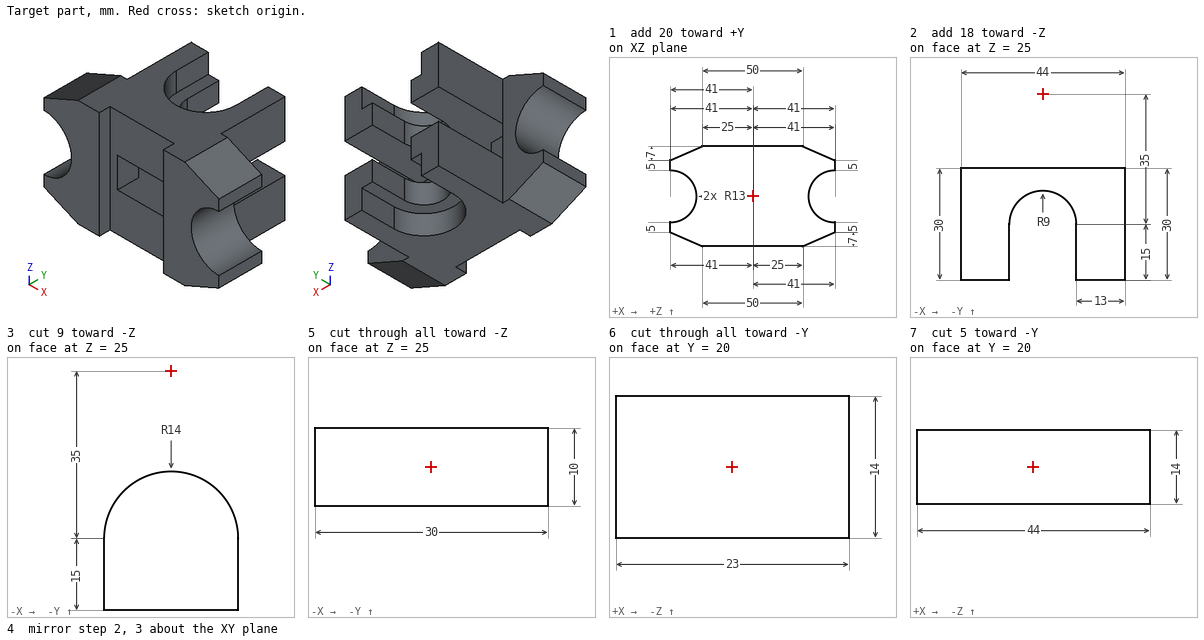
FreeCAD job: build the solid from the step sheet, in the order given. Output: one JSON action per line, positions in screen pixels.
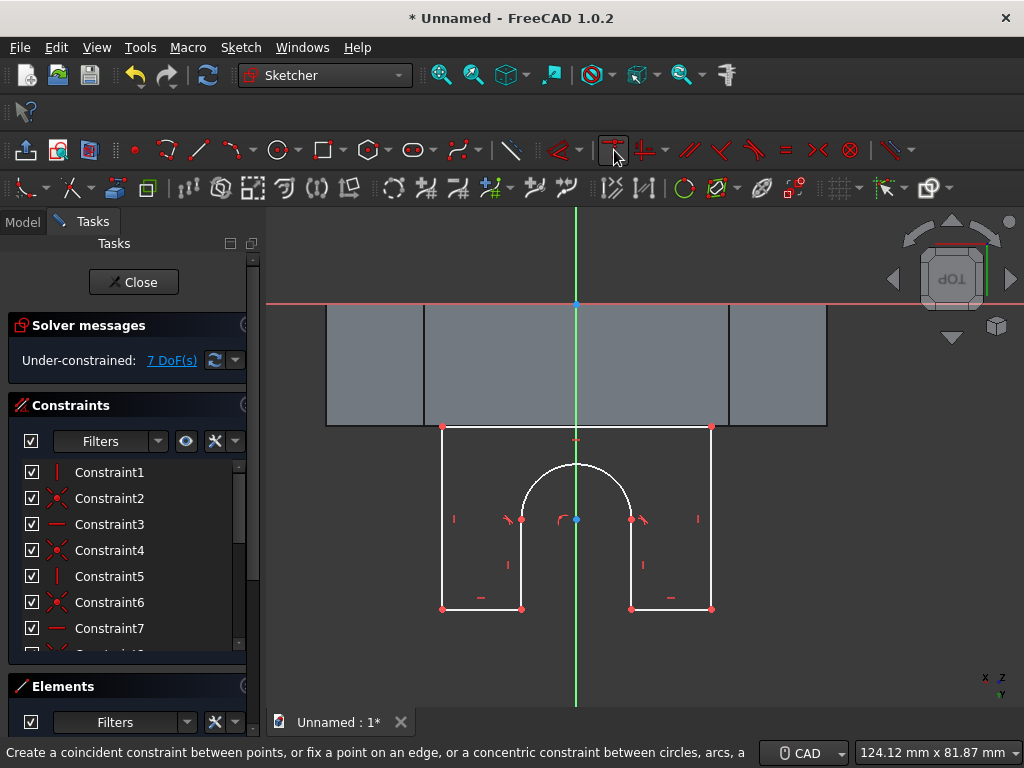
{"action": "left_click", "coordinate": [558, 150]}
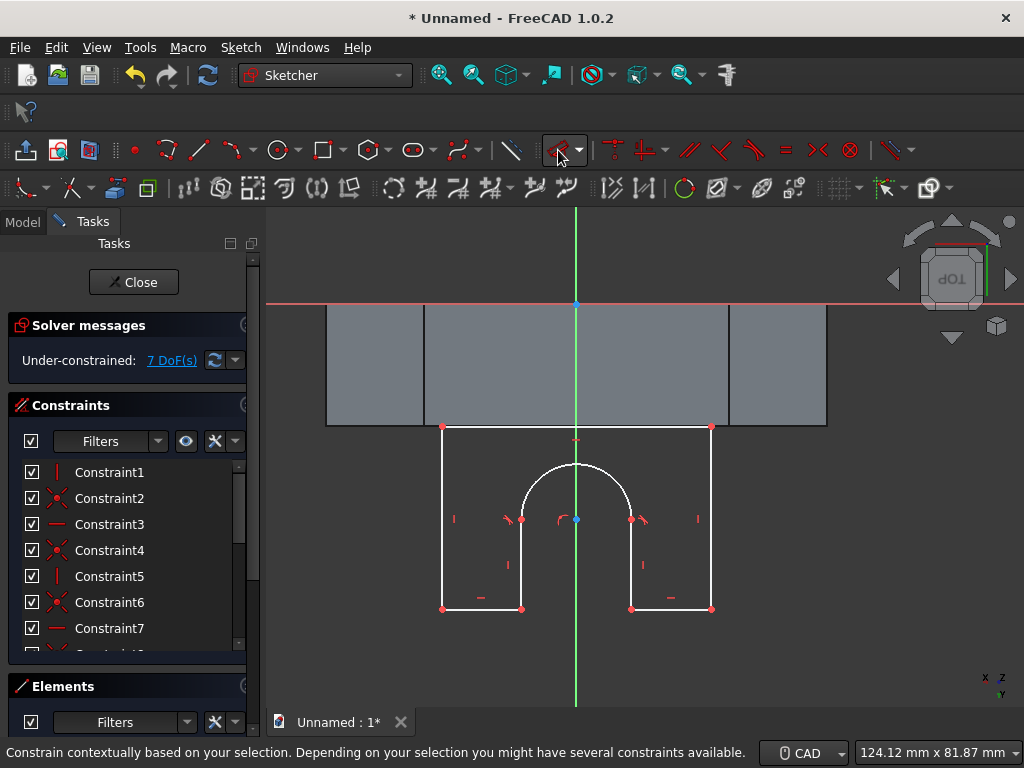
{"action": "left_click", "coordinate": [609, 475]}
{"action": "left_click", "coordinate": [628, 449]}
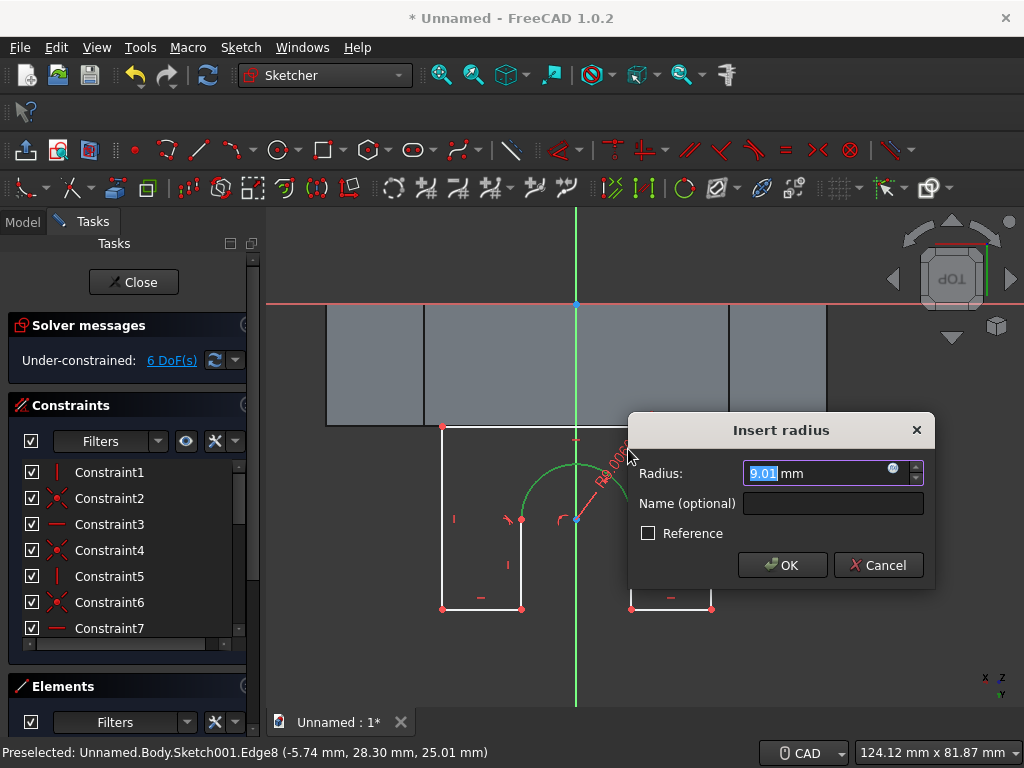
{"action": "type", "text": "9"}
{"action": "key", "text": "Return"}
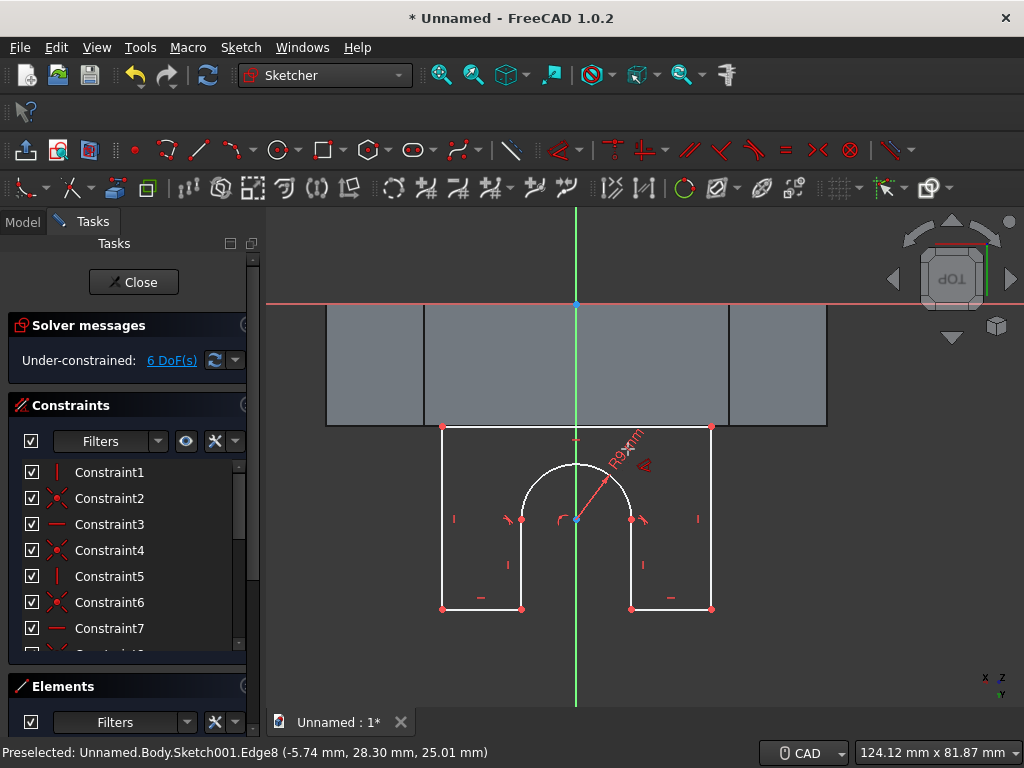
{"action": "left_click", "coordinate": [631, 547]}
{"action": "left_click", "coordinate": [665, 565]}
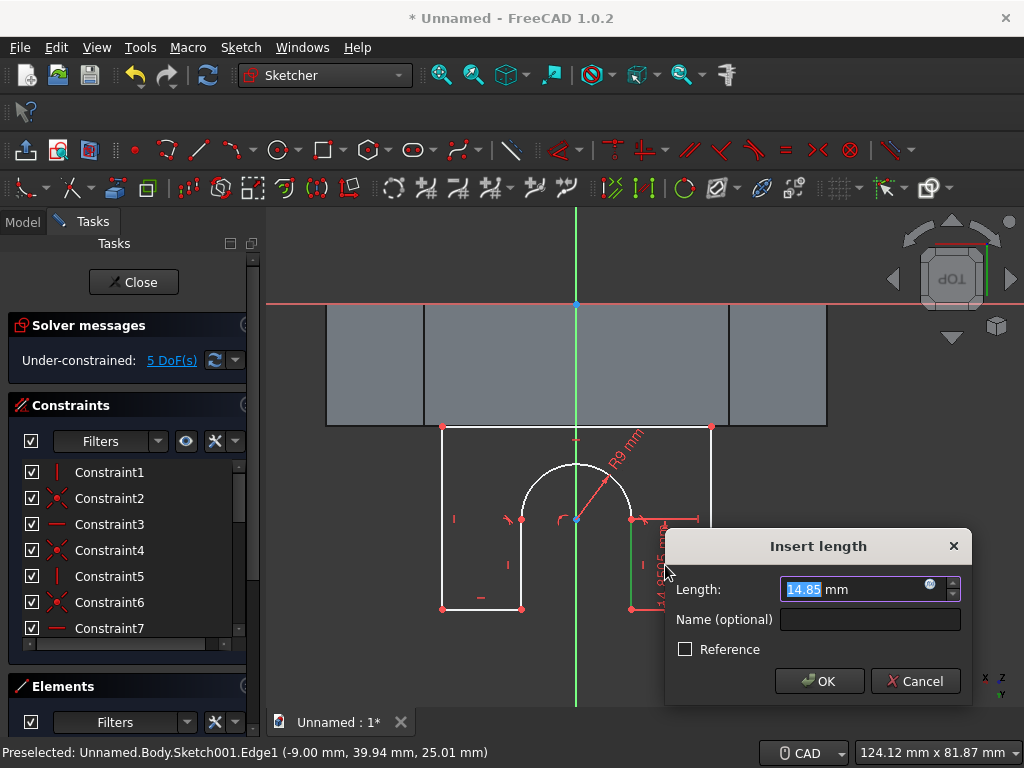
{"action": "type", "text": "15"}
{"action": "key", "text": "Return"}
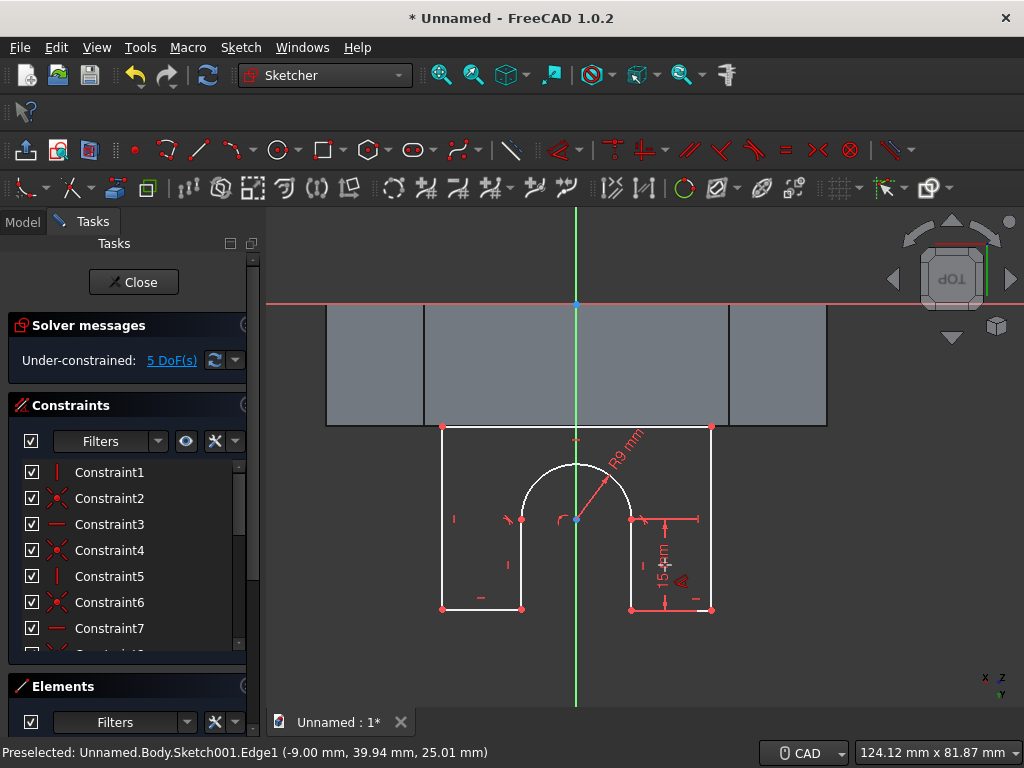
{"action": "left_click", "coordinate": [655, 611]}
{"action": "left_click", "coordinate": [671, 645]}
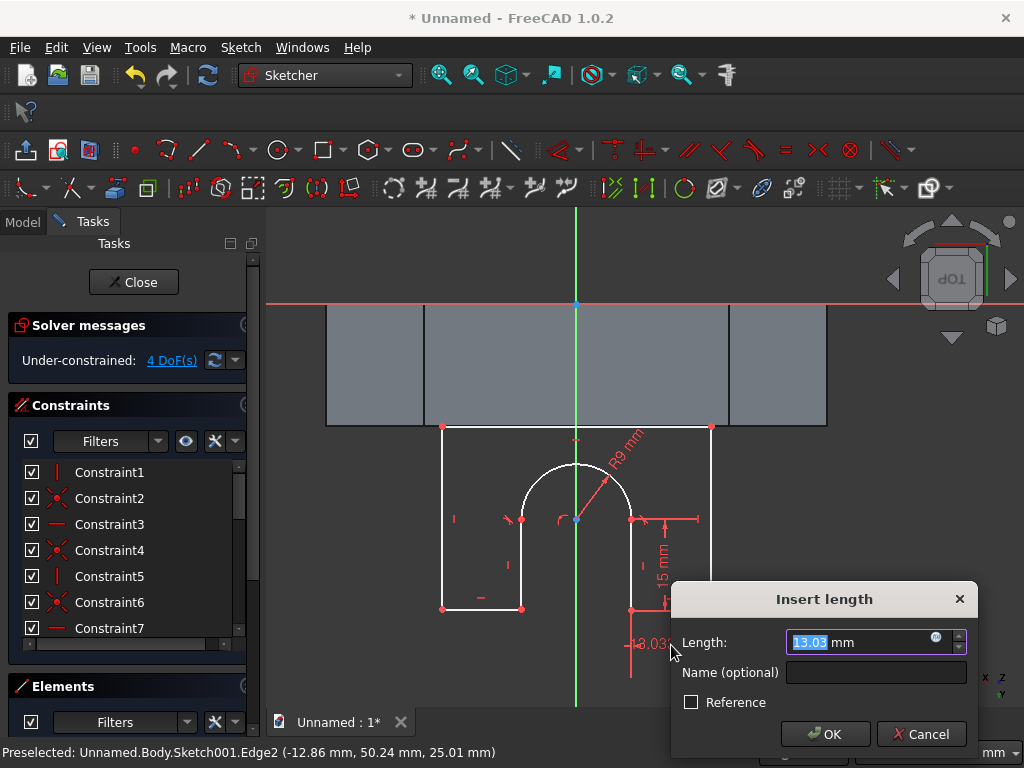
{"action": "type", "text": "13"}
{"action": "key", "text": "Return"}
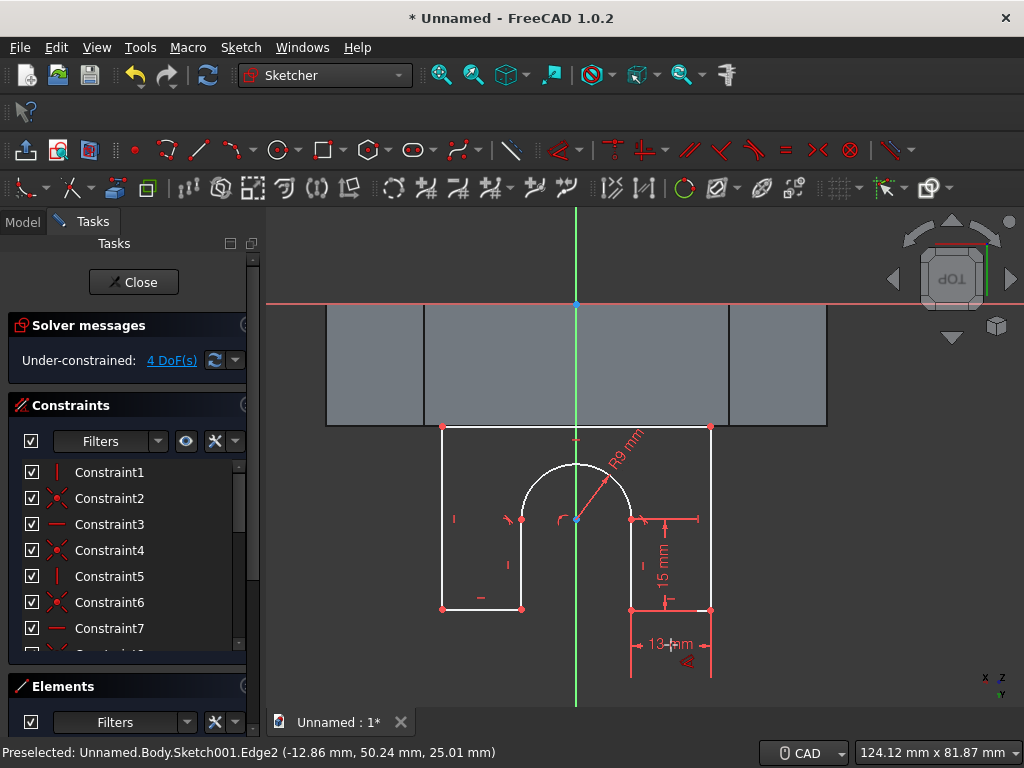
{"action": "left_click", "coordinate": [711, 556]}
{"action": "left_click", "coordinate": [745, 519]}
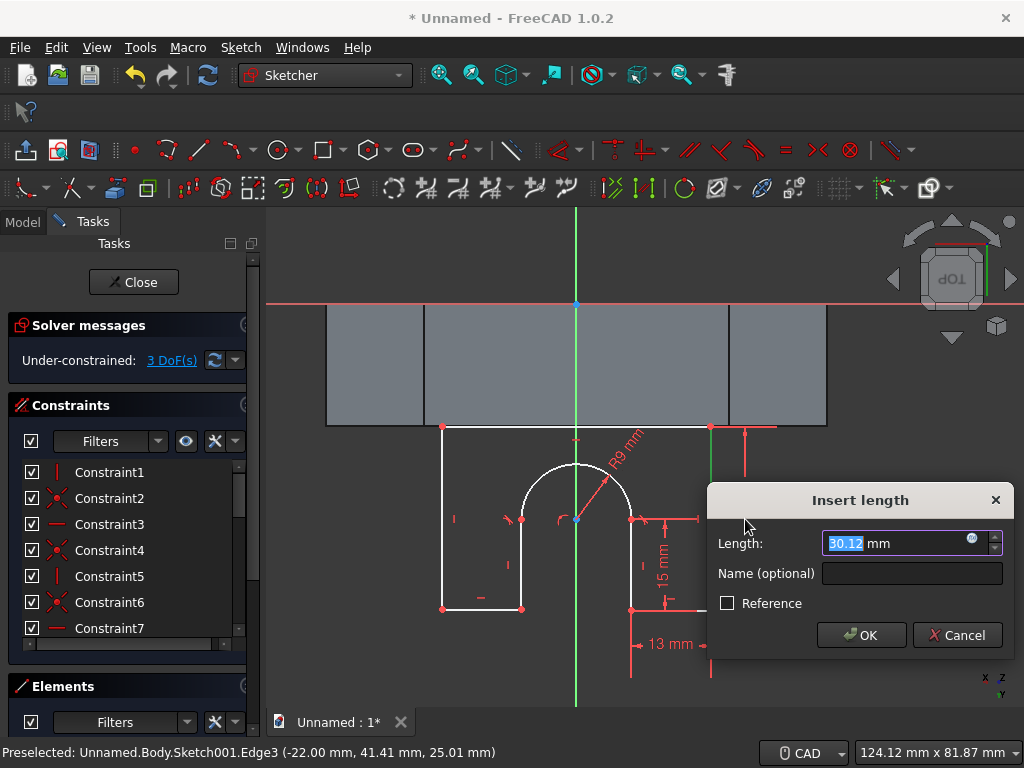
{"action": "type", "text": "30"}
{"action": "key", "text": "Return"}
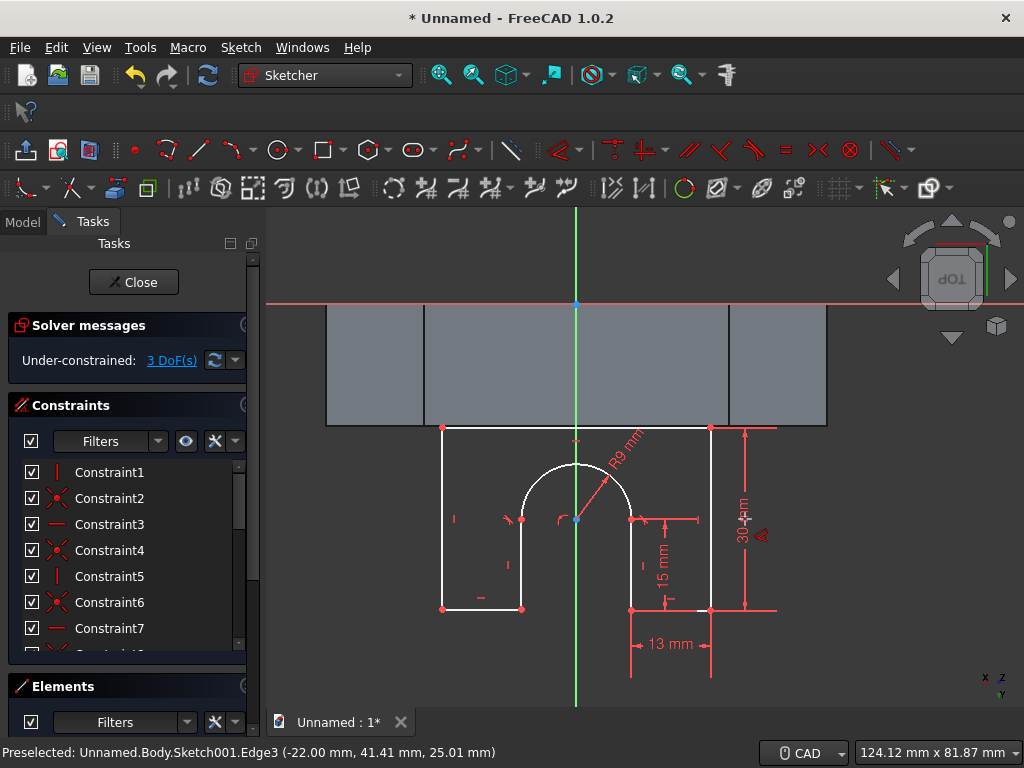
{"action": "left_click", "coordinate": [630, 428]}
{"action": "left_click", "coordinate": [515, 394]}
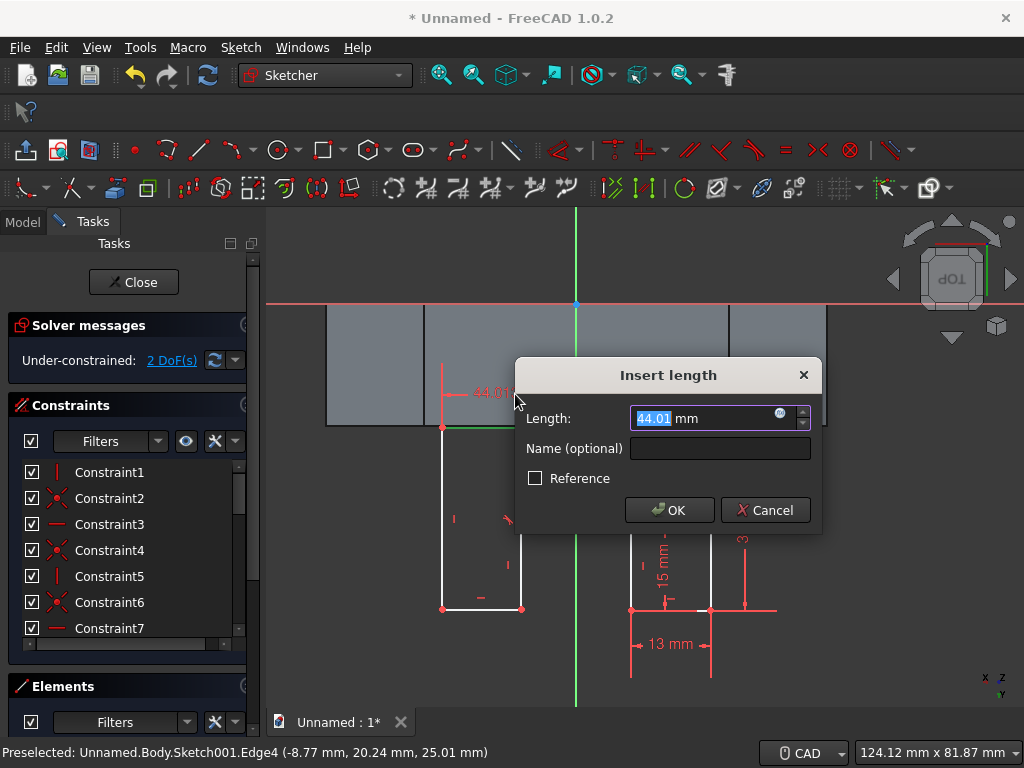
{"action": "type", "text": "44"}
{"action": "key", "text": "Return"}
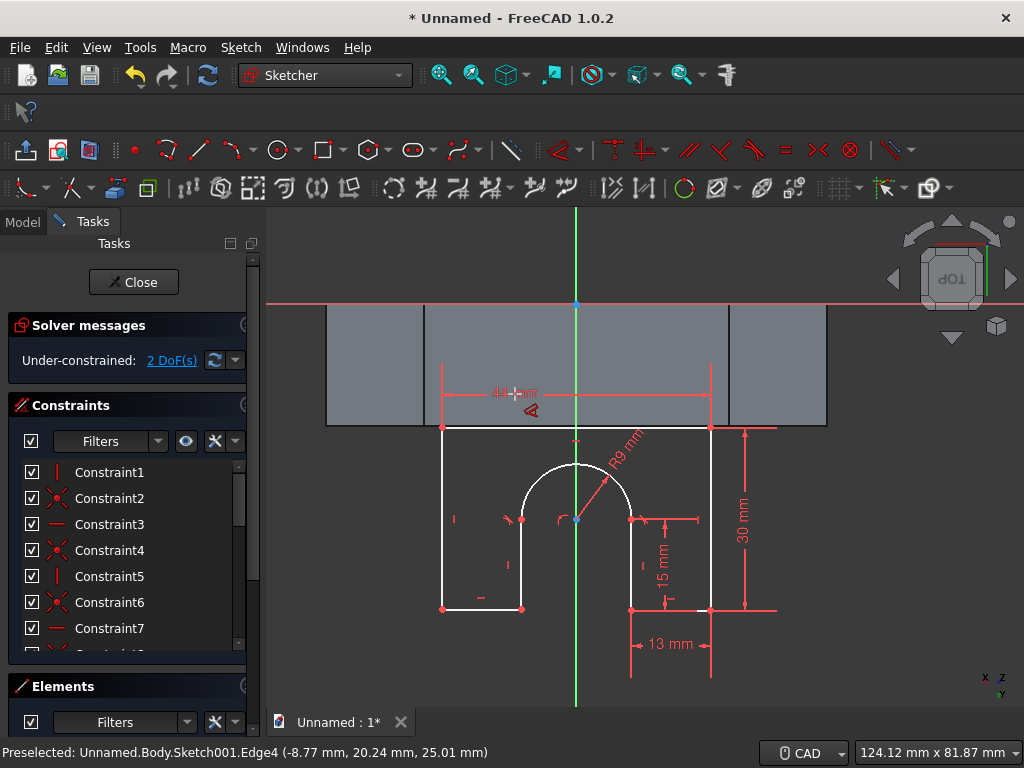
{"action": "left_click", "coordinate": [442, 482]}
{"action": "left_click", "coordinate": [408, 519]}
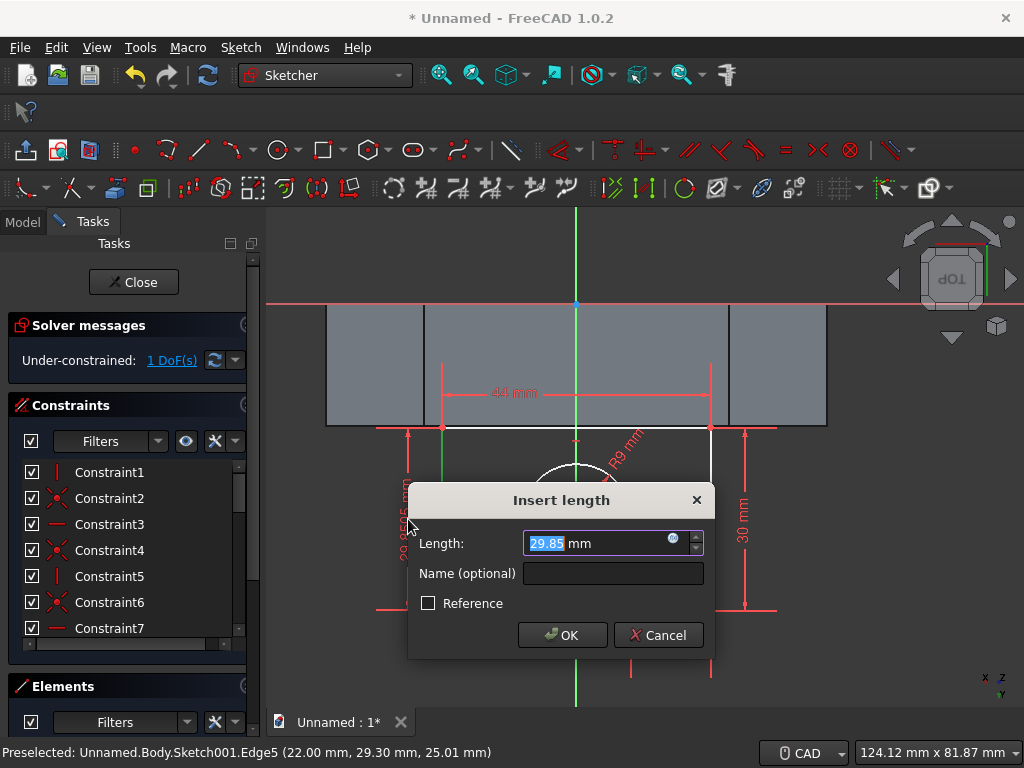
{"action": "type", "text": "30"}
{"action": "key", "text": "Return"}